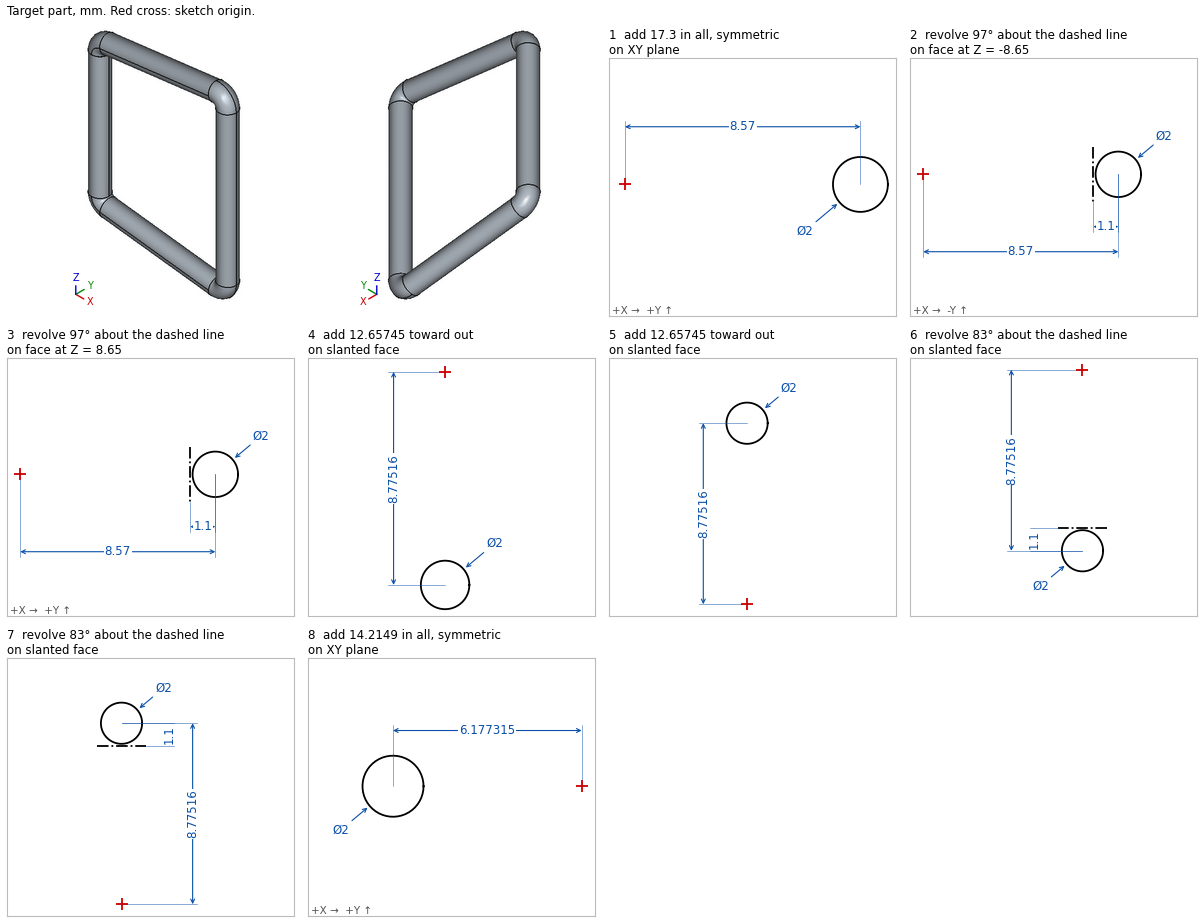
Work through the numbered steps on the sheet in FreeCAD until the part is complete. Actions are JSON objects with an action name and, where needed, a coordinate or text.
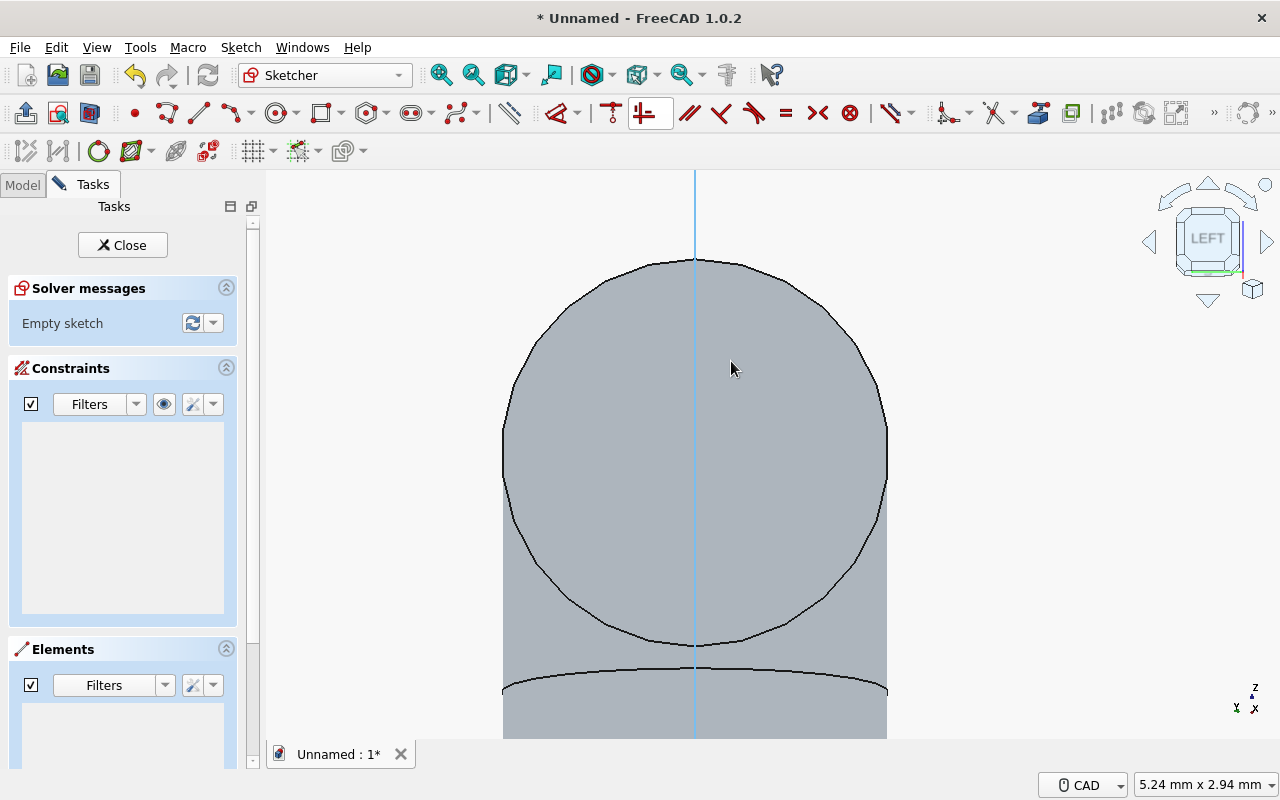
{"action": "left_click", "coordinate": [276, 114]}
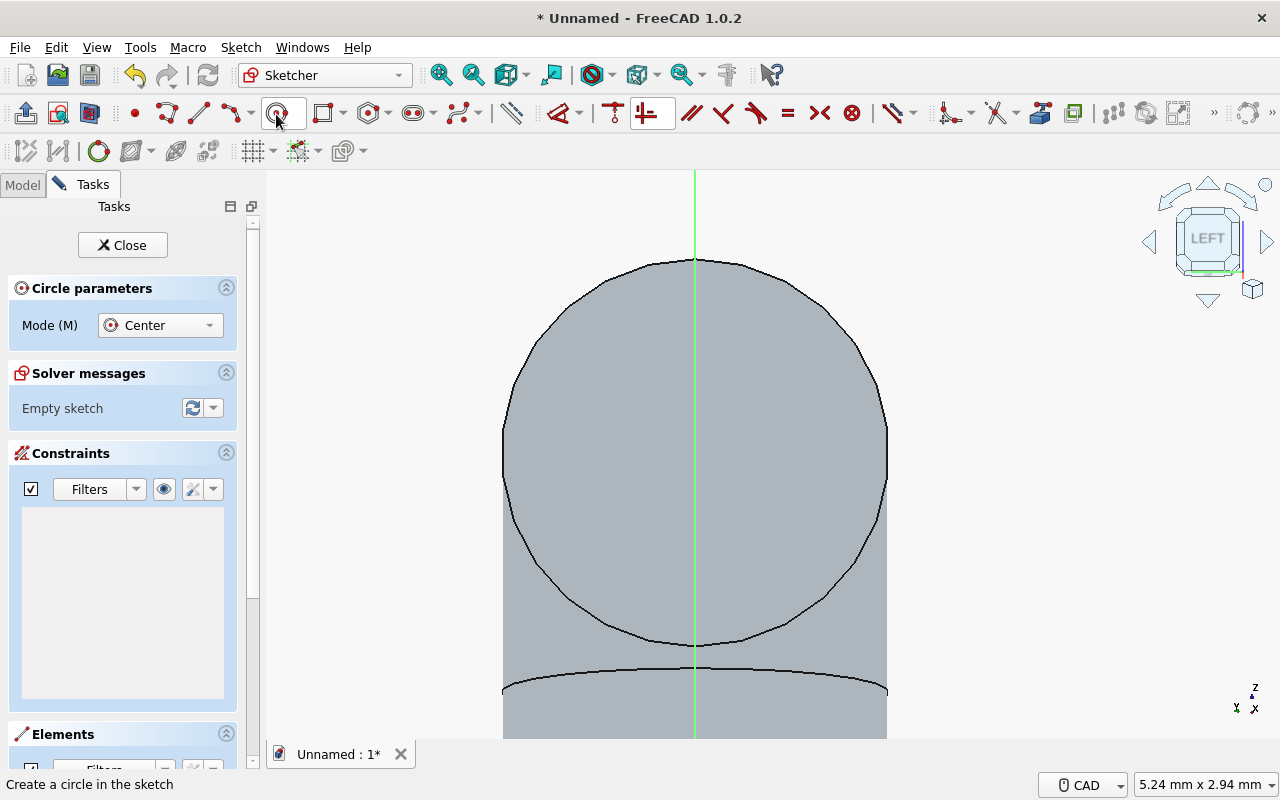
{"action": "left_click", "coordinate": [695, 453]}
{"action": "mouse_move", "coordinate": [832, 316]}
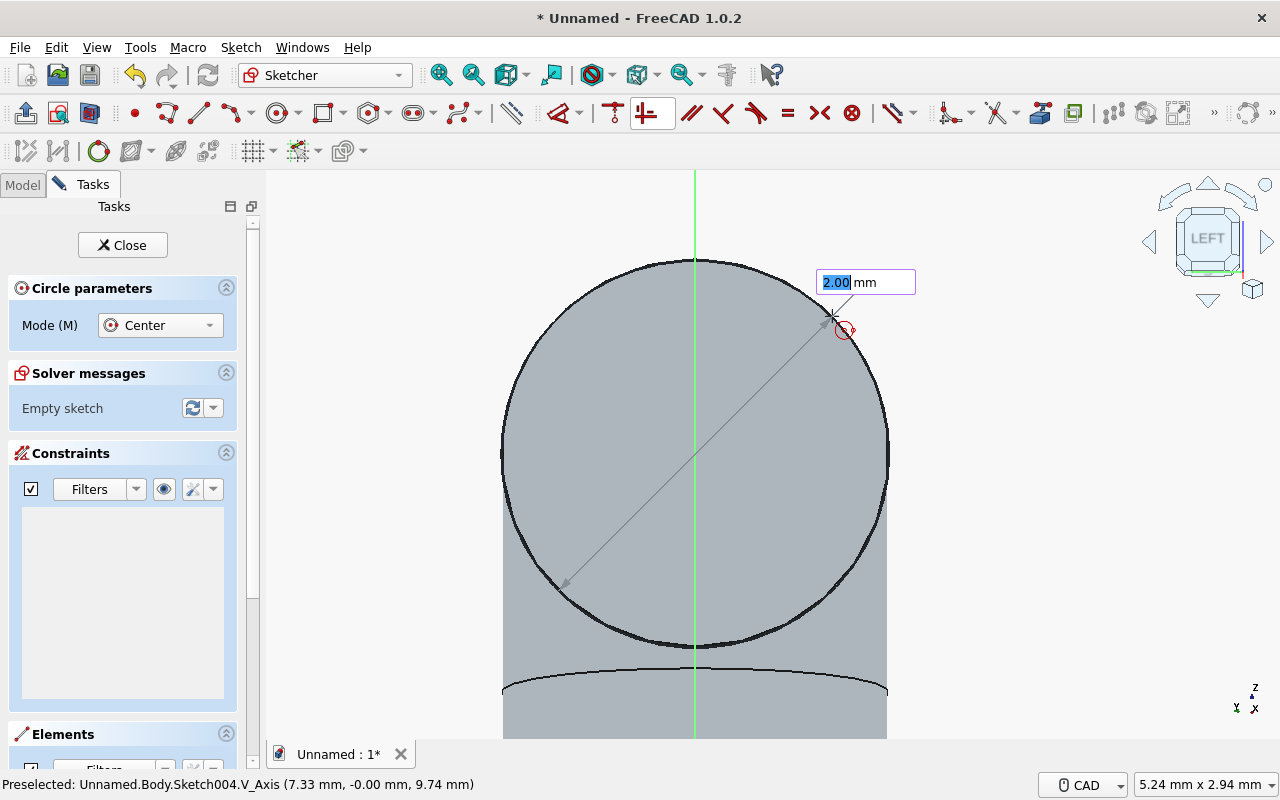
{"action": "type", "text": "2"}
{"action": "key", "text": "Return"}
{"action": "key", "text": "Escape"}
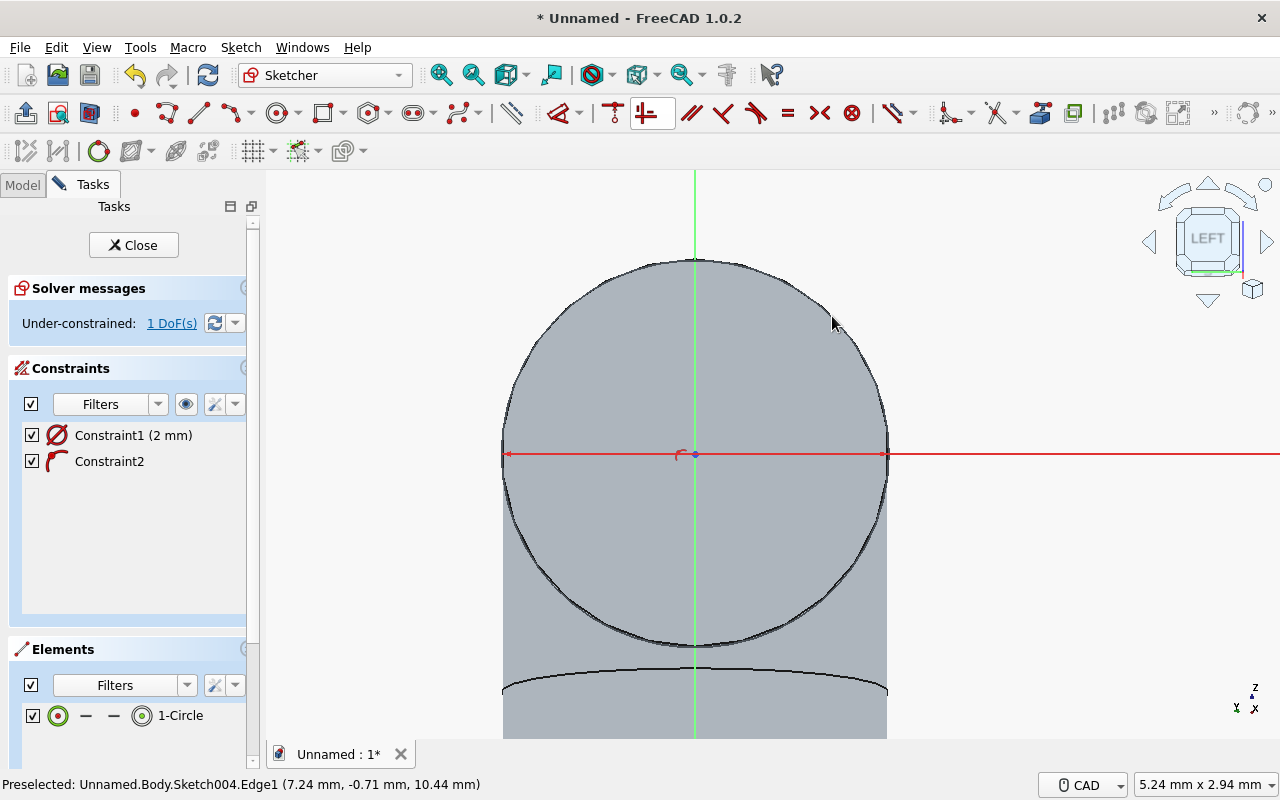
{"action": "left_click", "coordinate": [558, 114]}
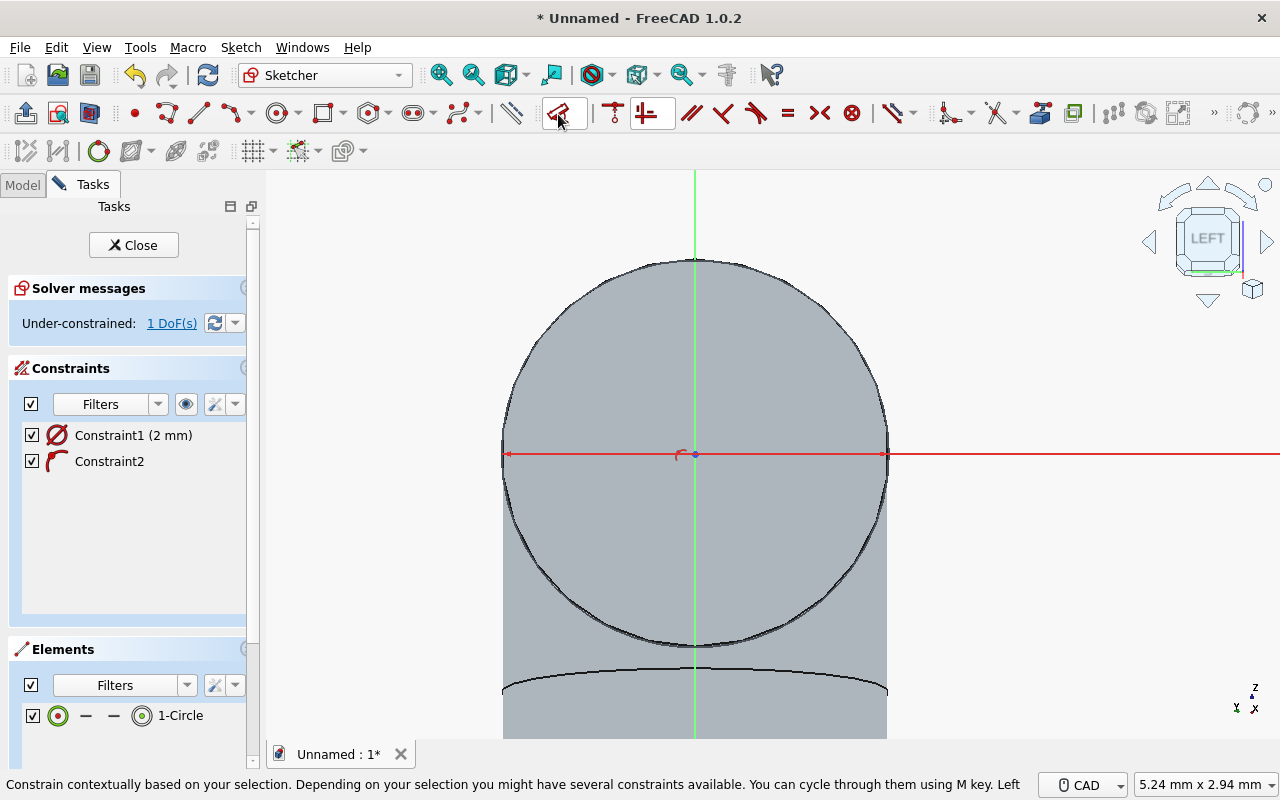
{"action": "left_click", "coordinate": [695, 454]}
{"action": "left_click", "coordinate": [661, 583]}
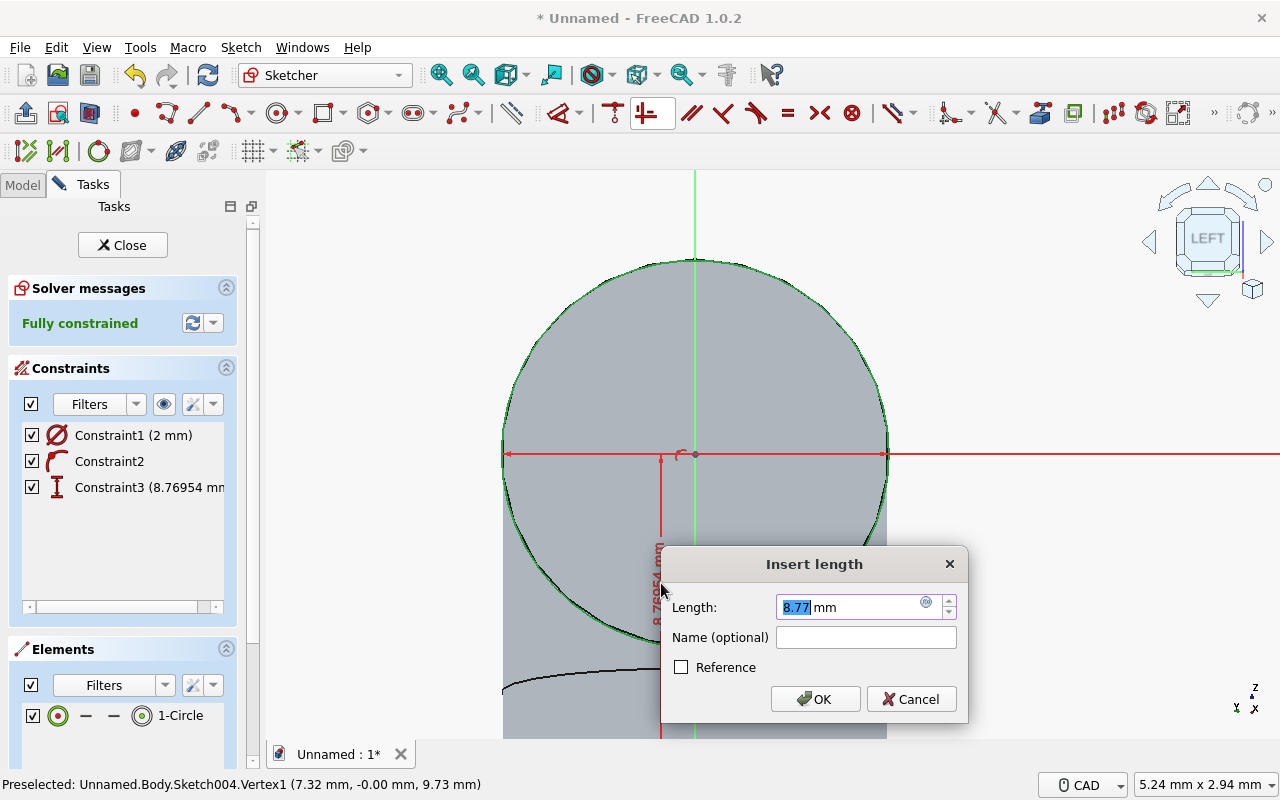
{"action": "type", "text": "8.77516"}
{"action": "key", "text": "Return"}
{"action": "key", "text": "Escape"}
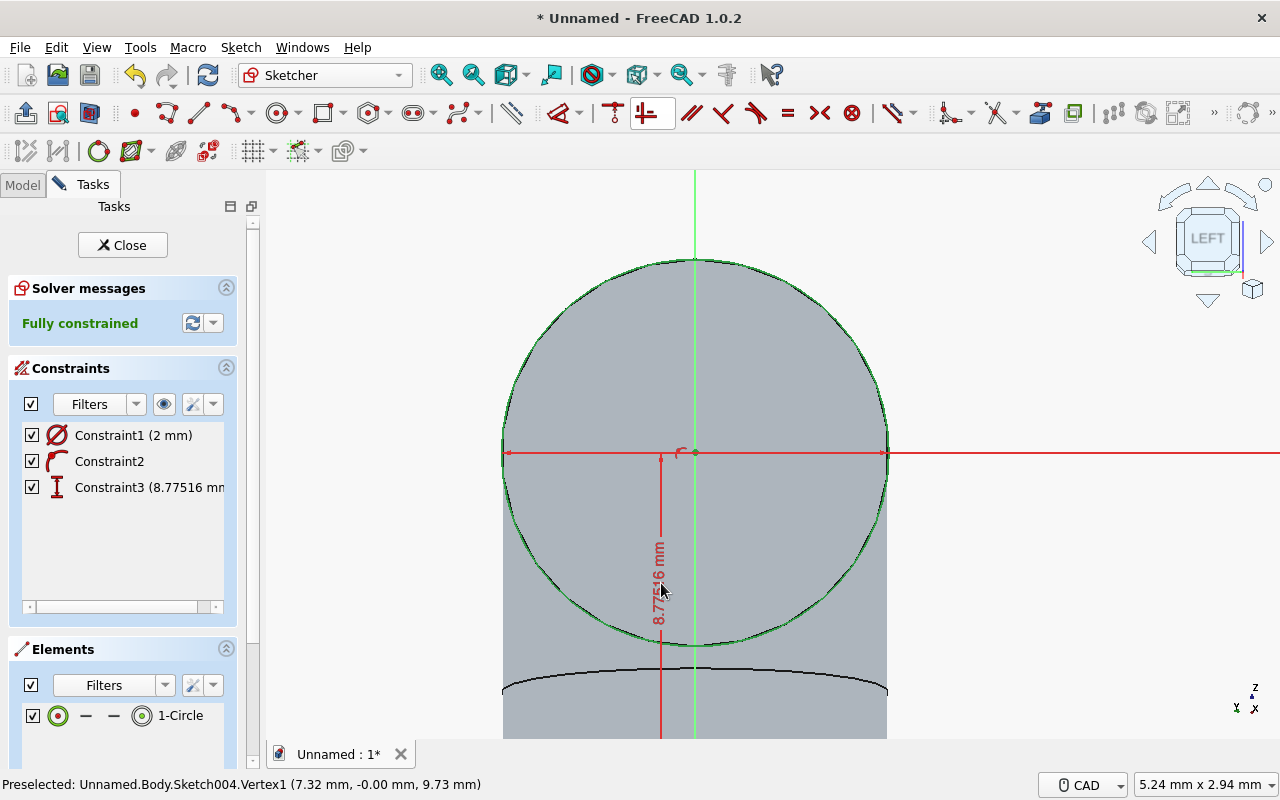
{"action": "left_click", "coordinate": [123, 245]}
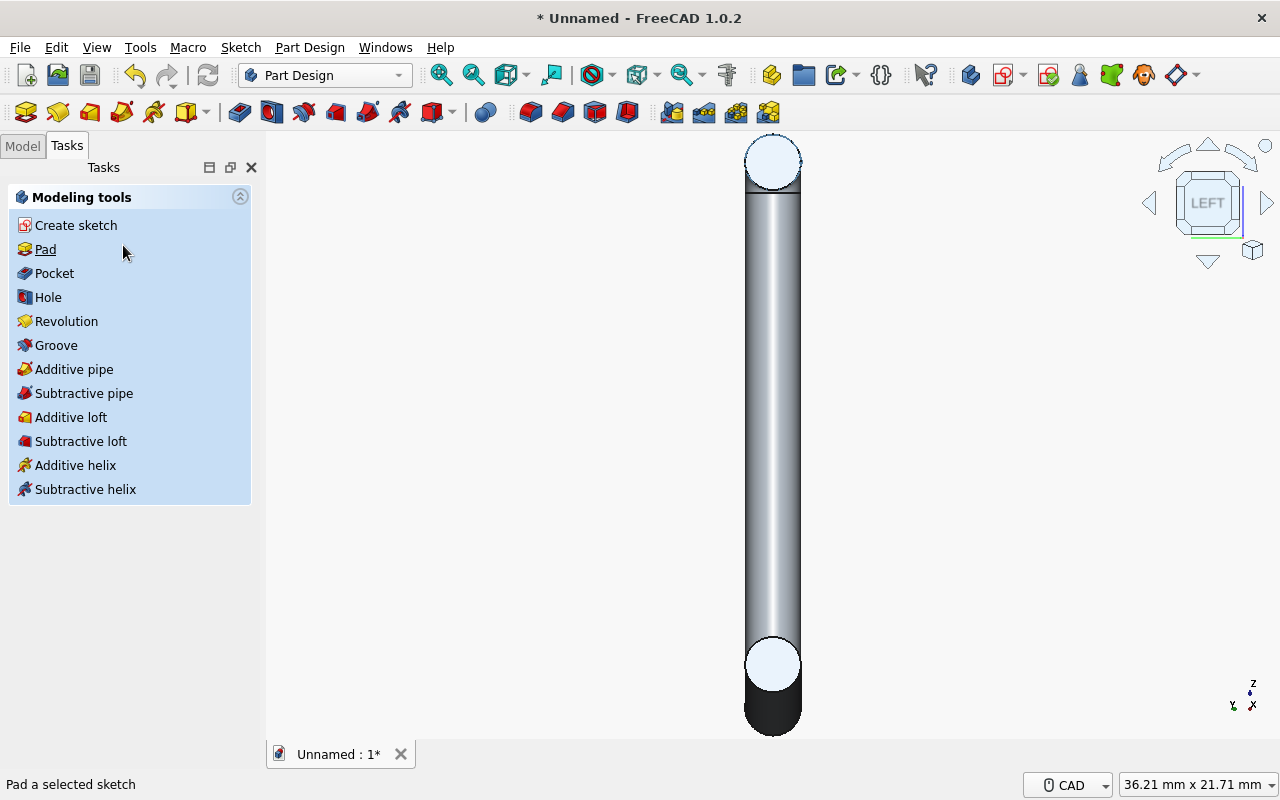
{"action": "left_click", "coordinate": [26, 112]}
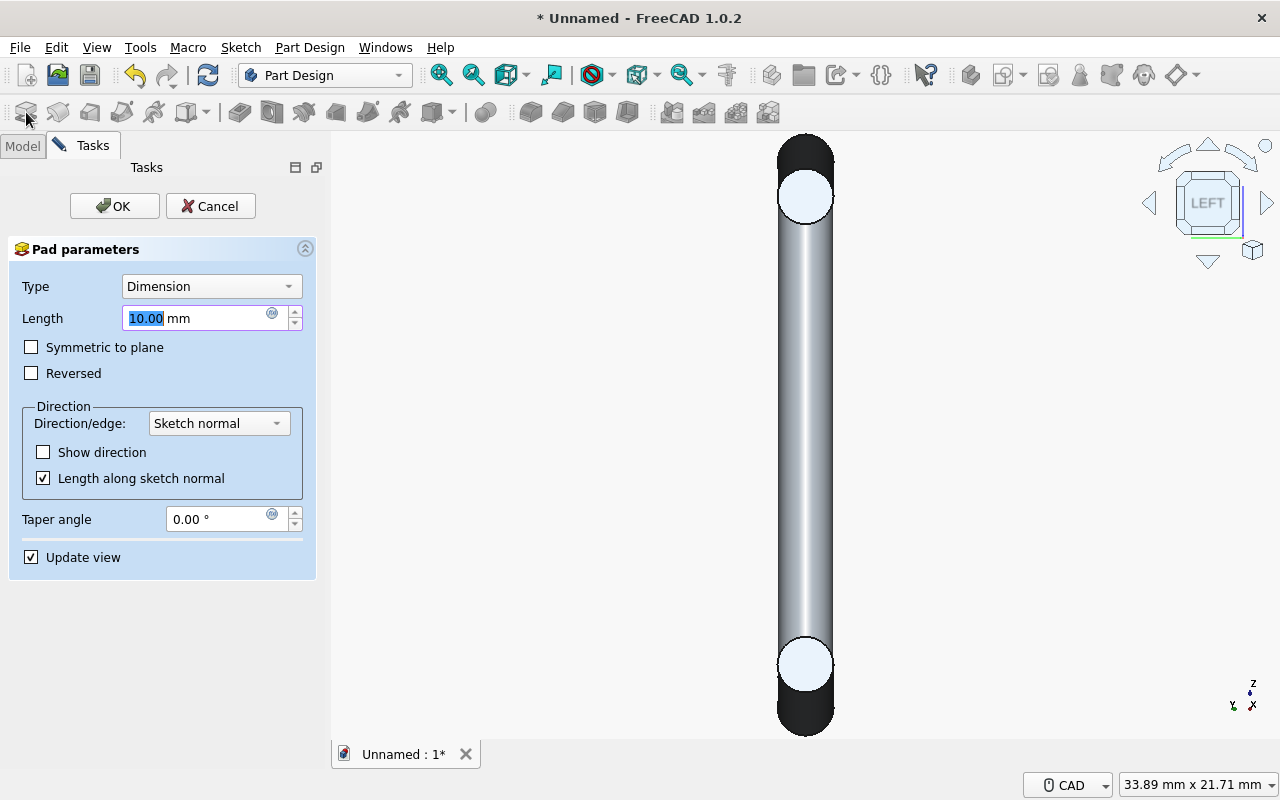
{"action": "type", "text": "12.65745"}
{"action": "key", "text": "Tab"}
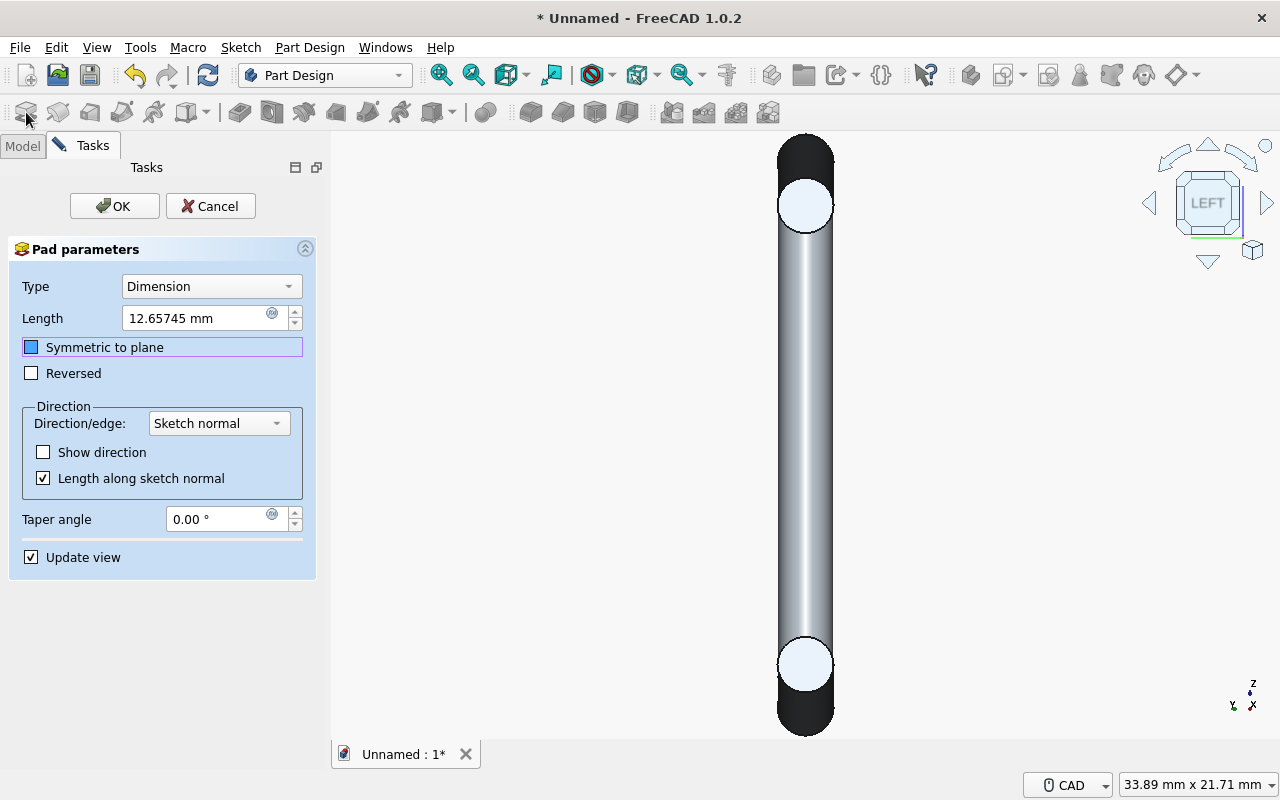
{"action": "left_click", "coordinate": [115, 206]}